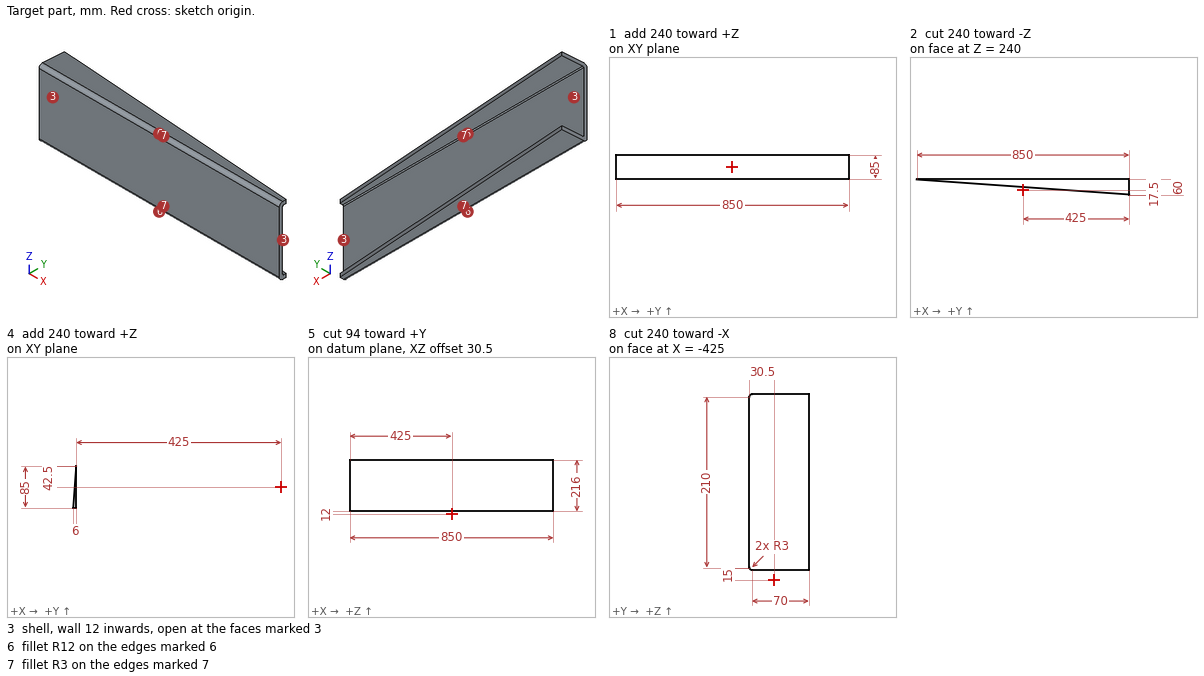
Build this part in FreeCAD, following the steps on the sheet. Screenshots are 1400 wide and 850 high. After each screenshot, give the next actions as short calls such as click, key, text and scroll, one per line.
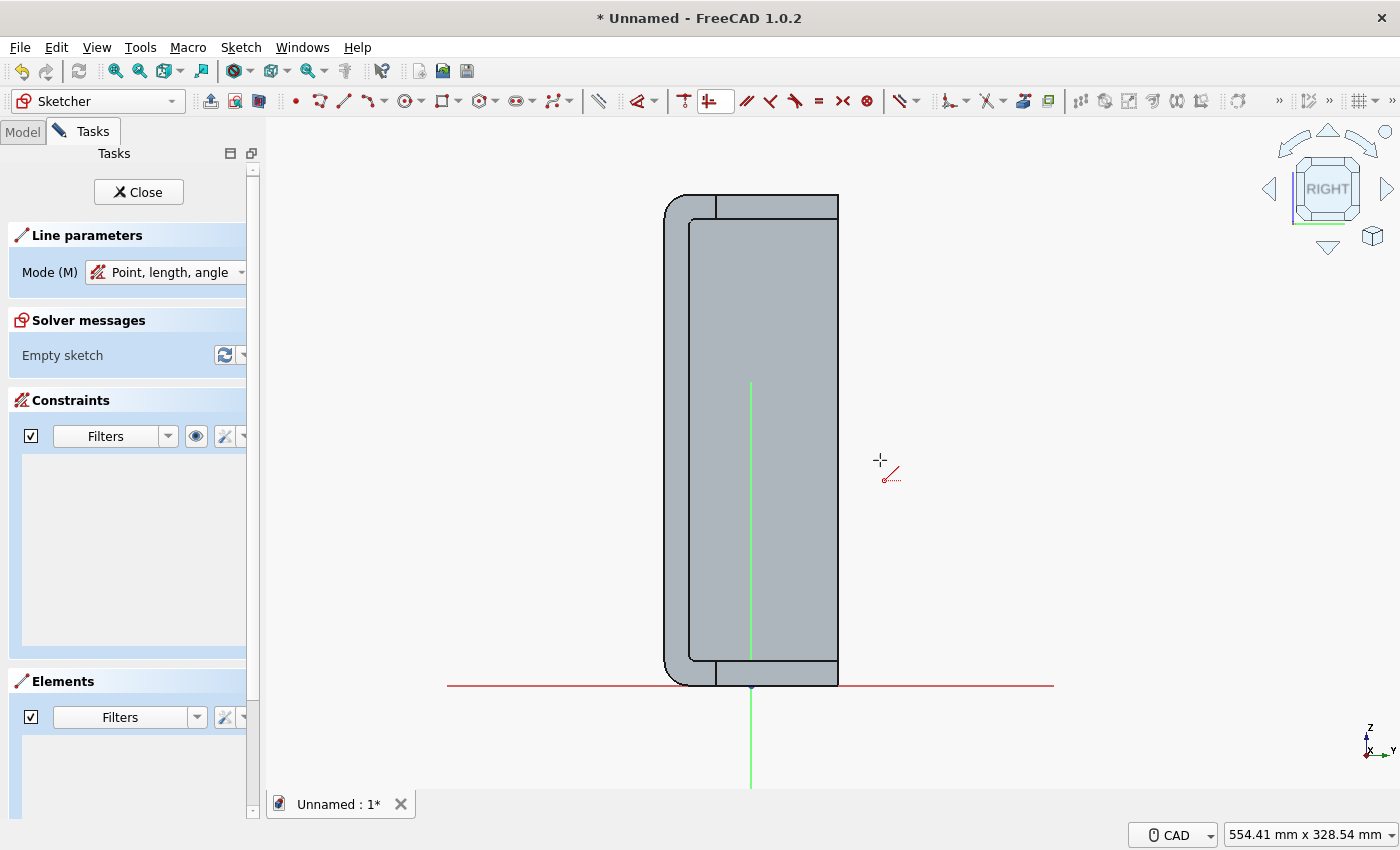
click(689, 225)
click(689, 655)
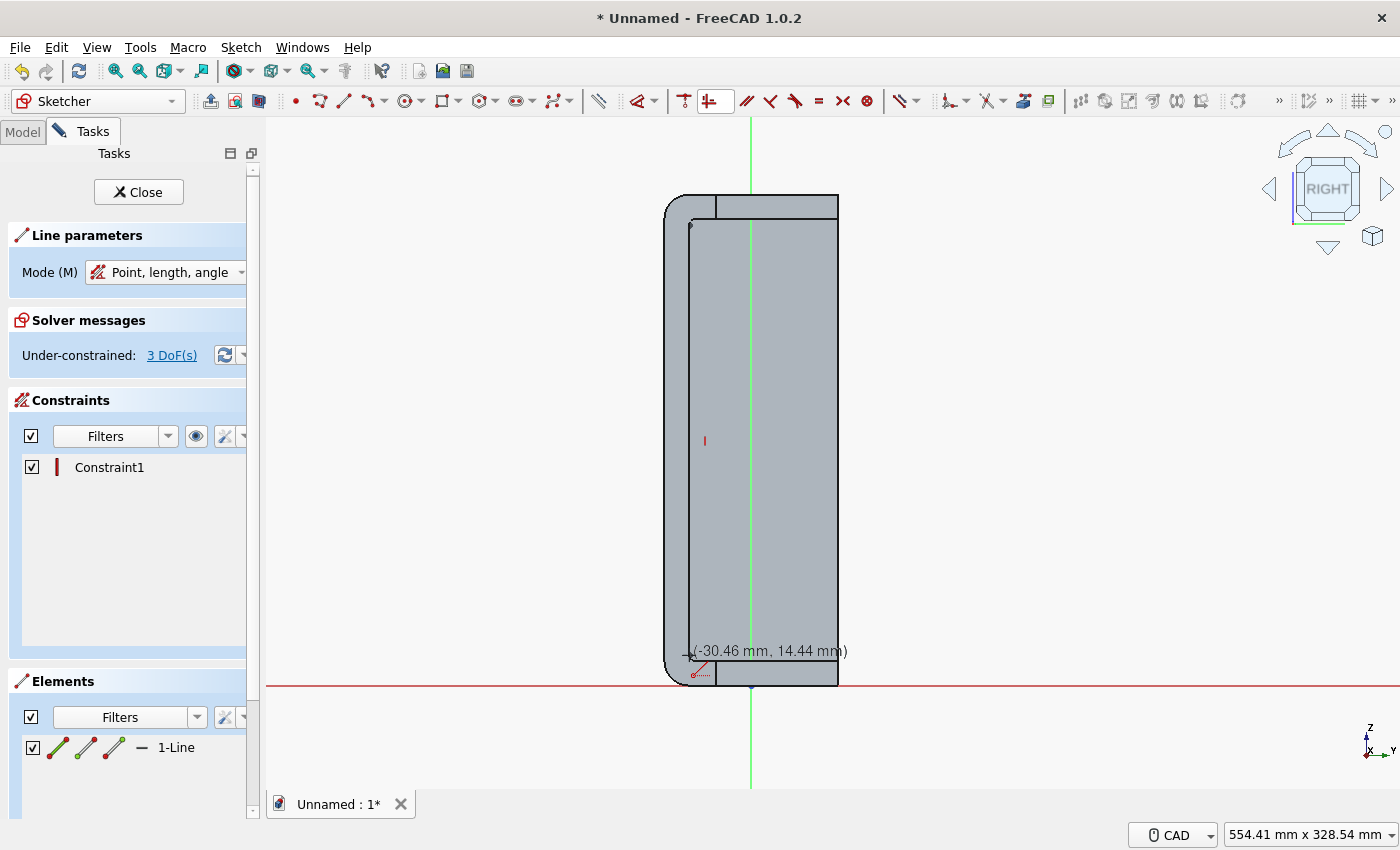
key(g)
key(m)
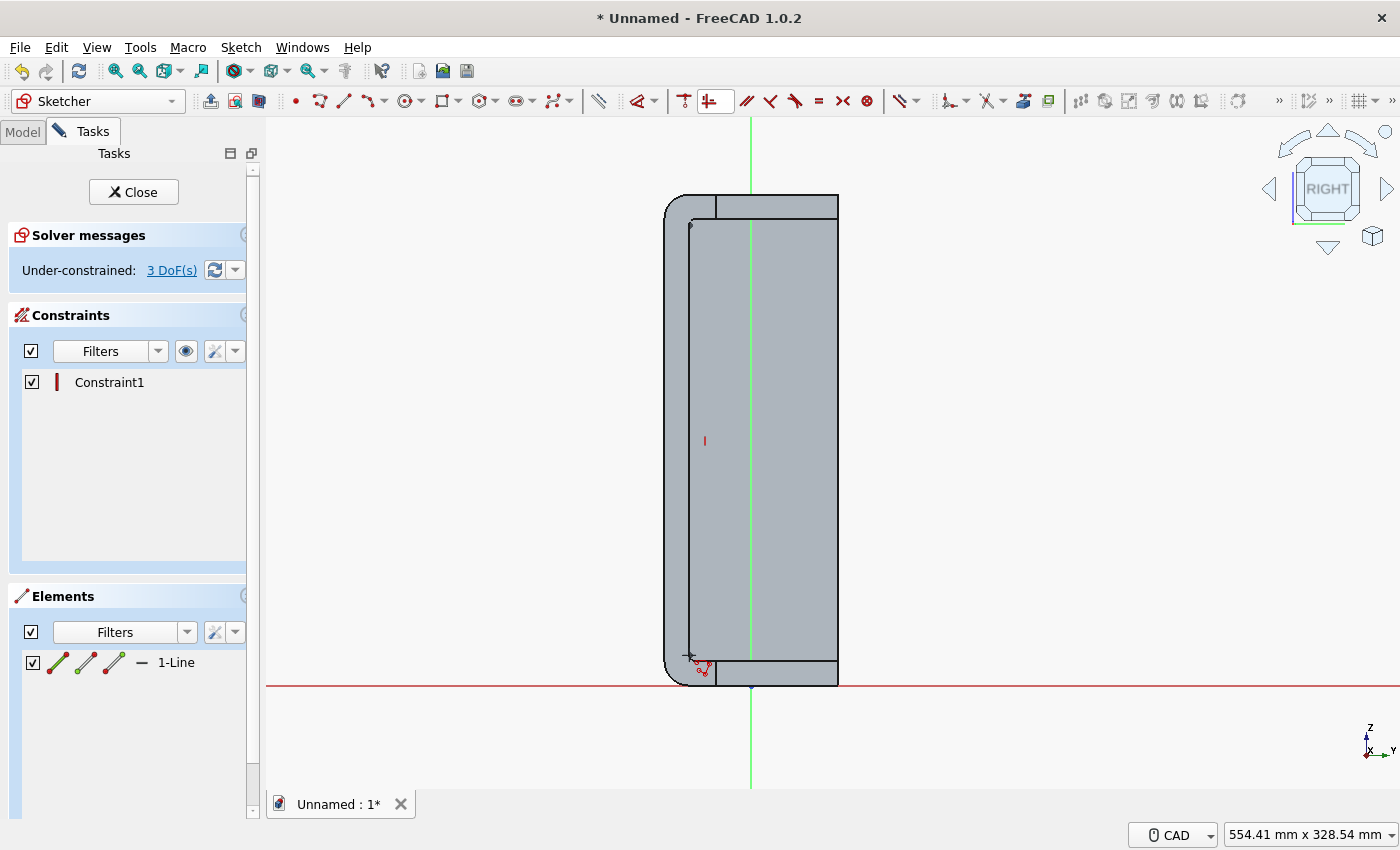
scroll(695, 661, up, 4)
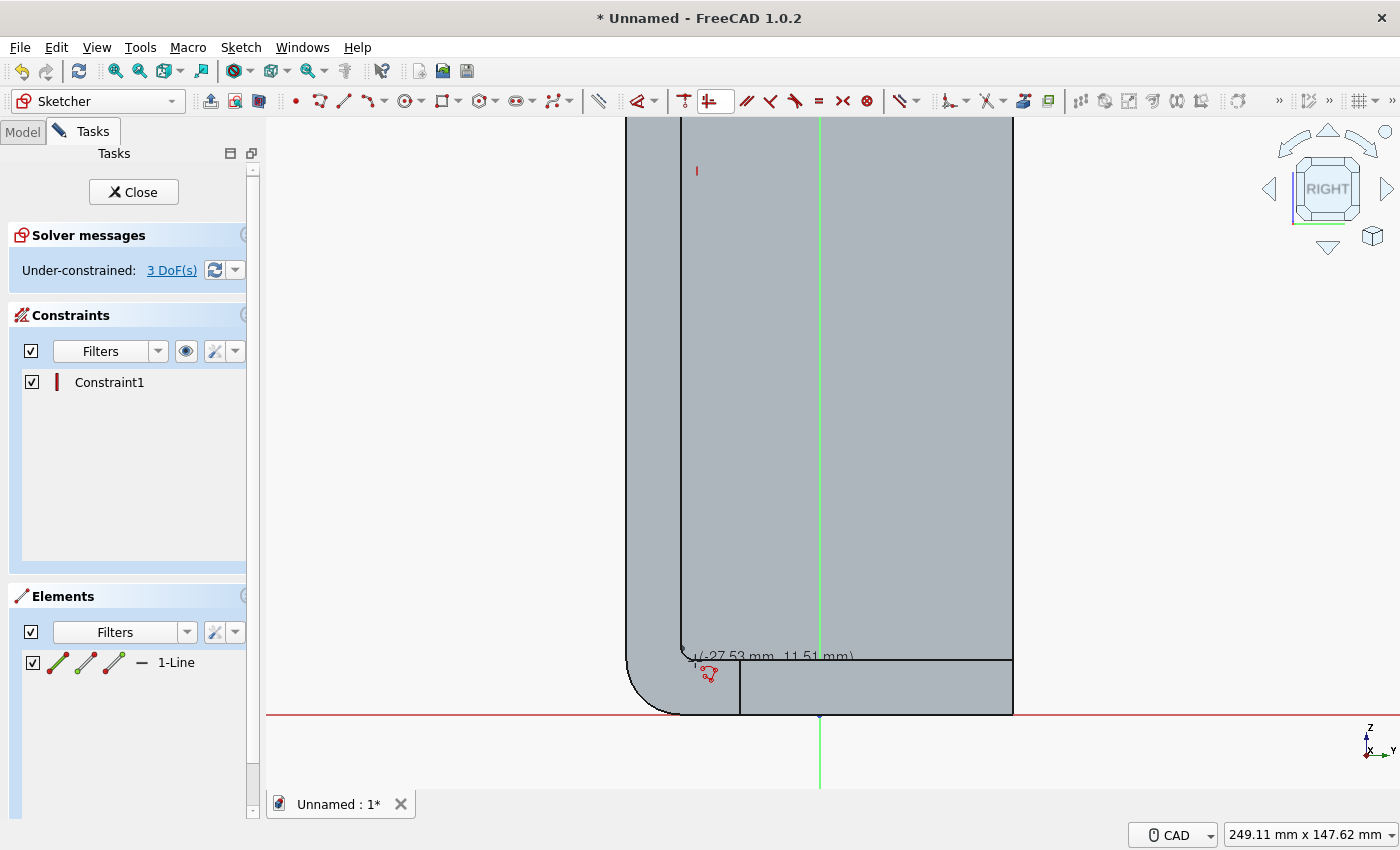
click(695, 660)
click(1013, 660)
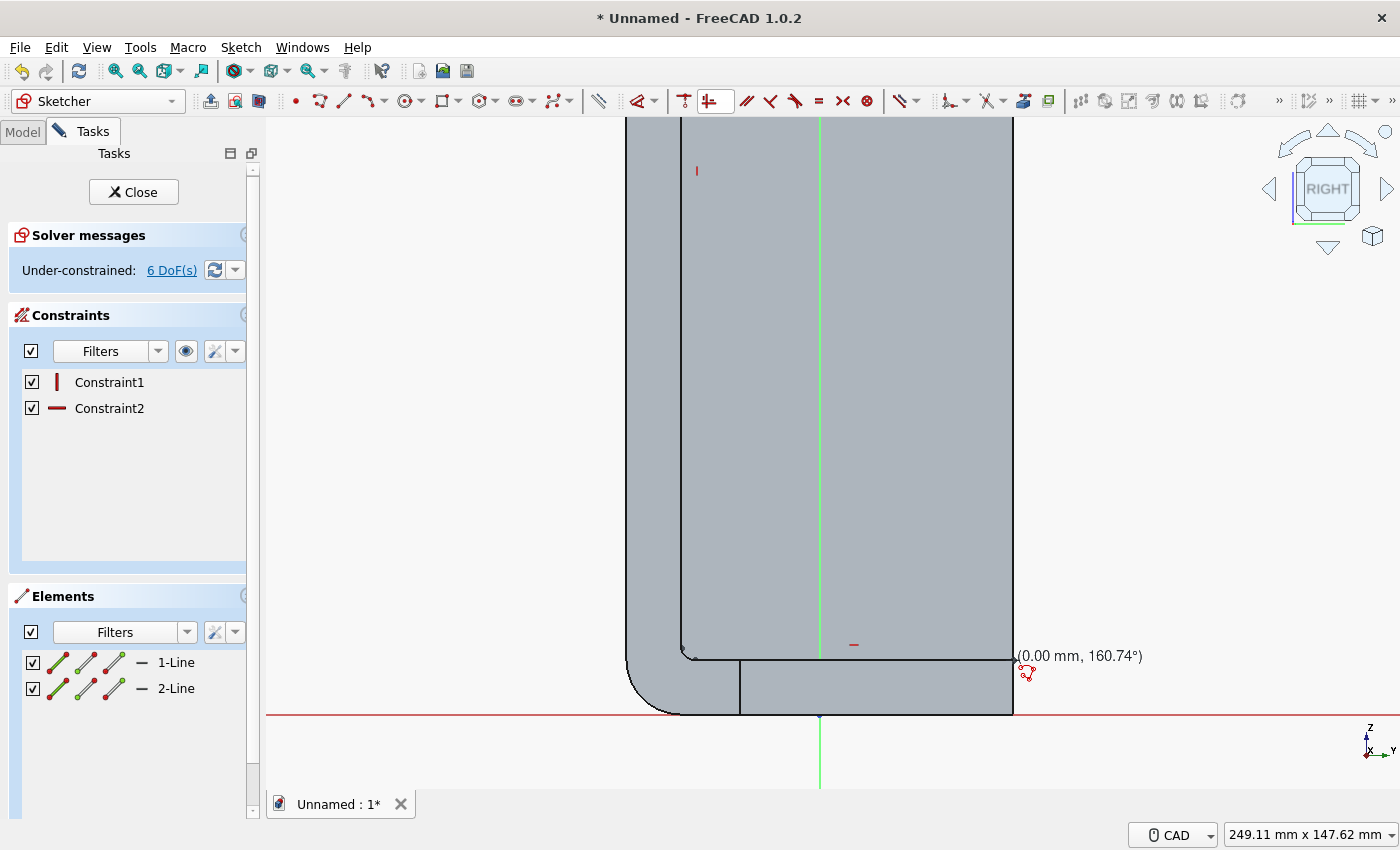
scroll(697, 663, down, 4)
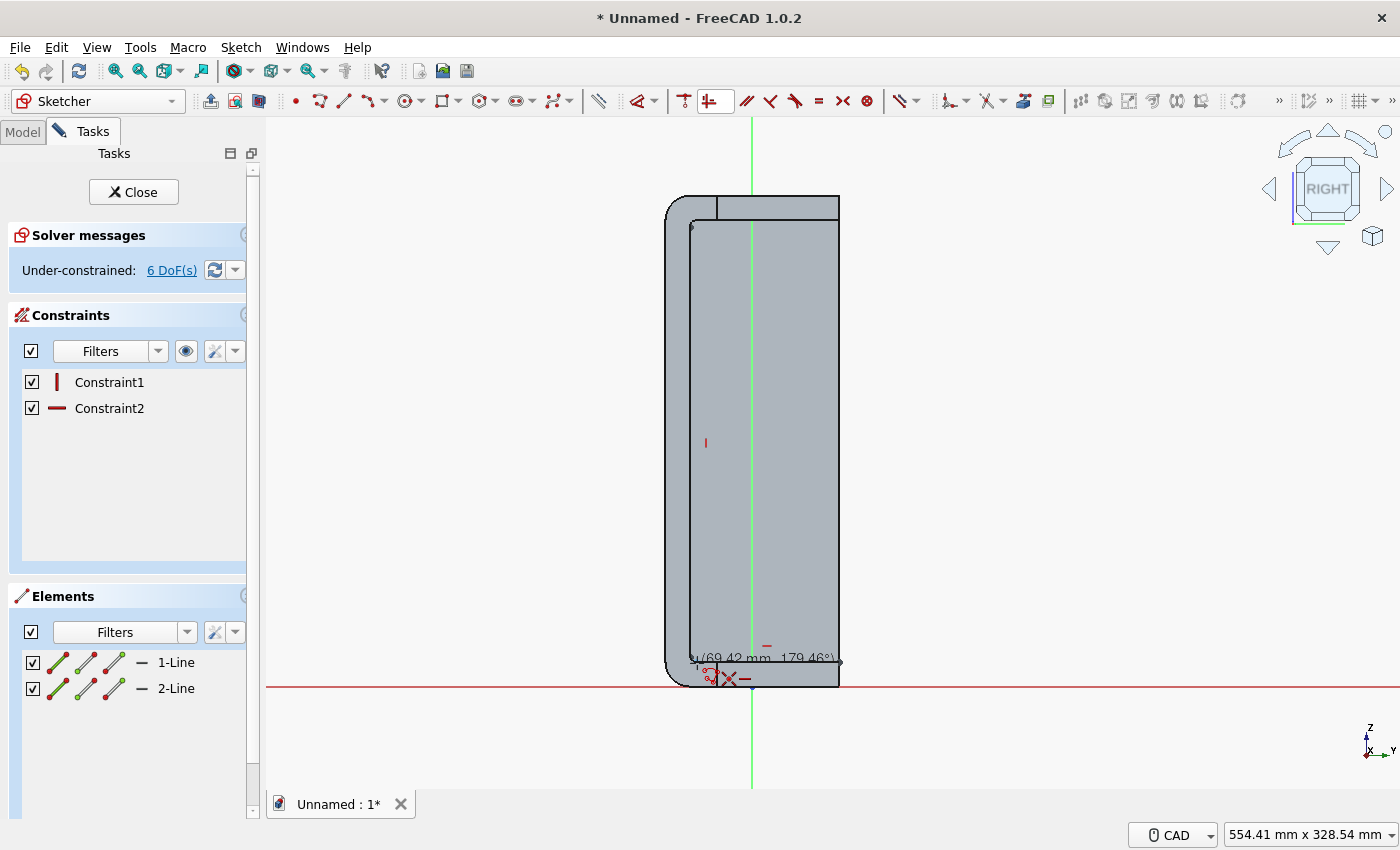
click(839, 220)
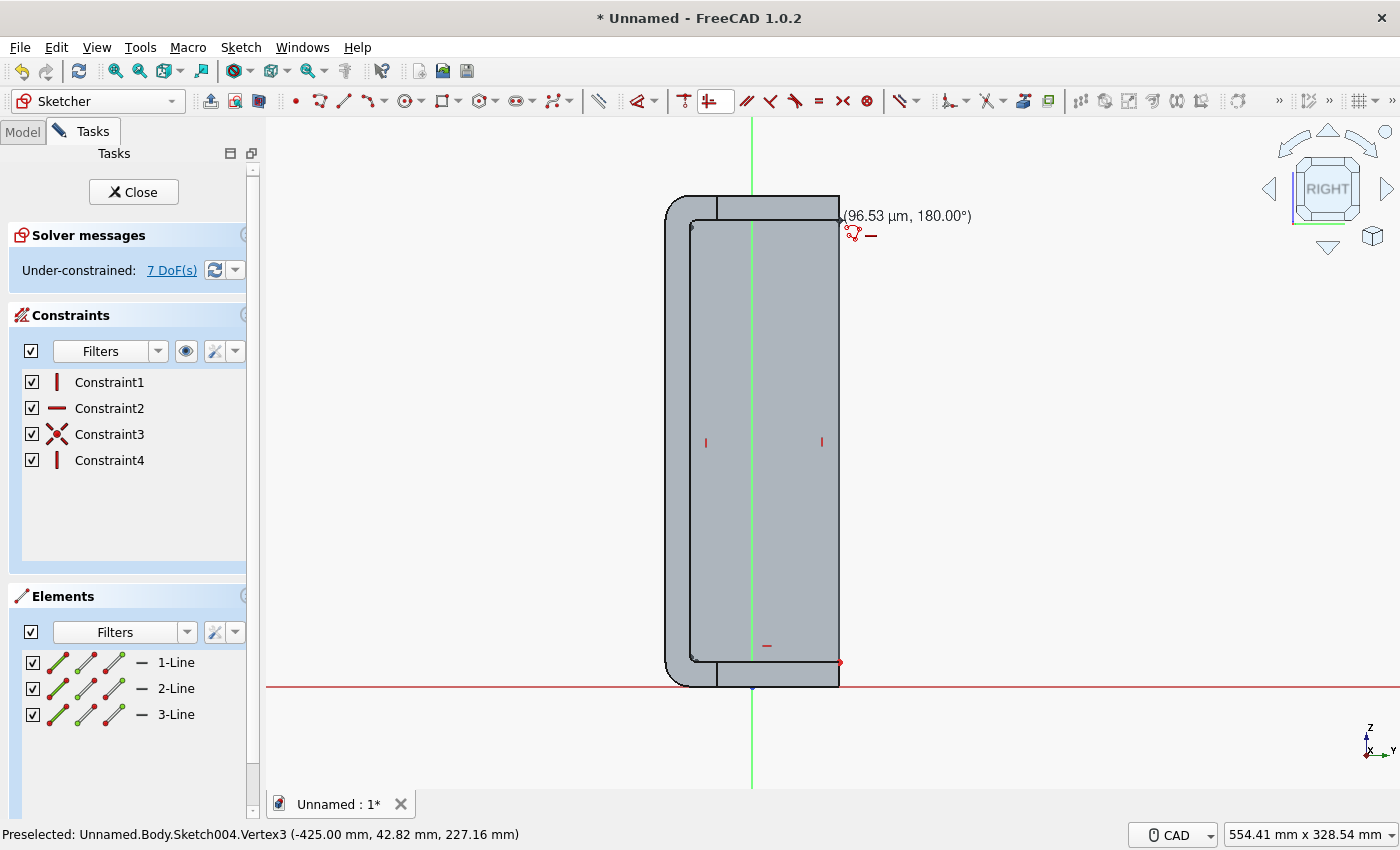
scroll(696, 220, up, 4)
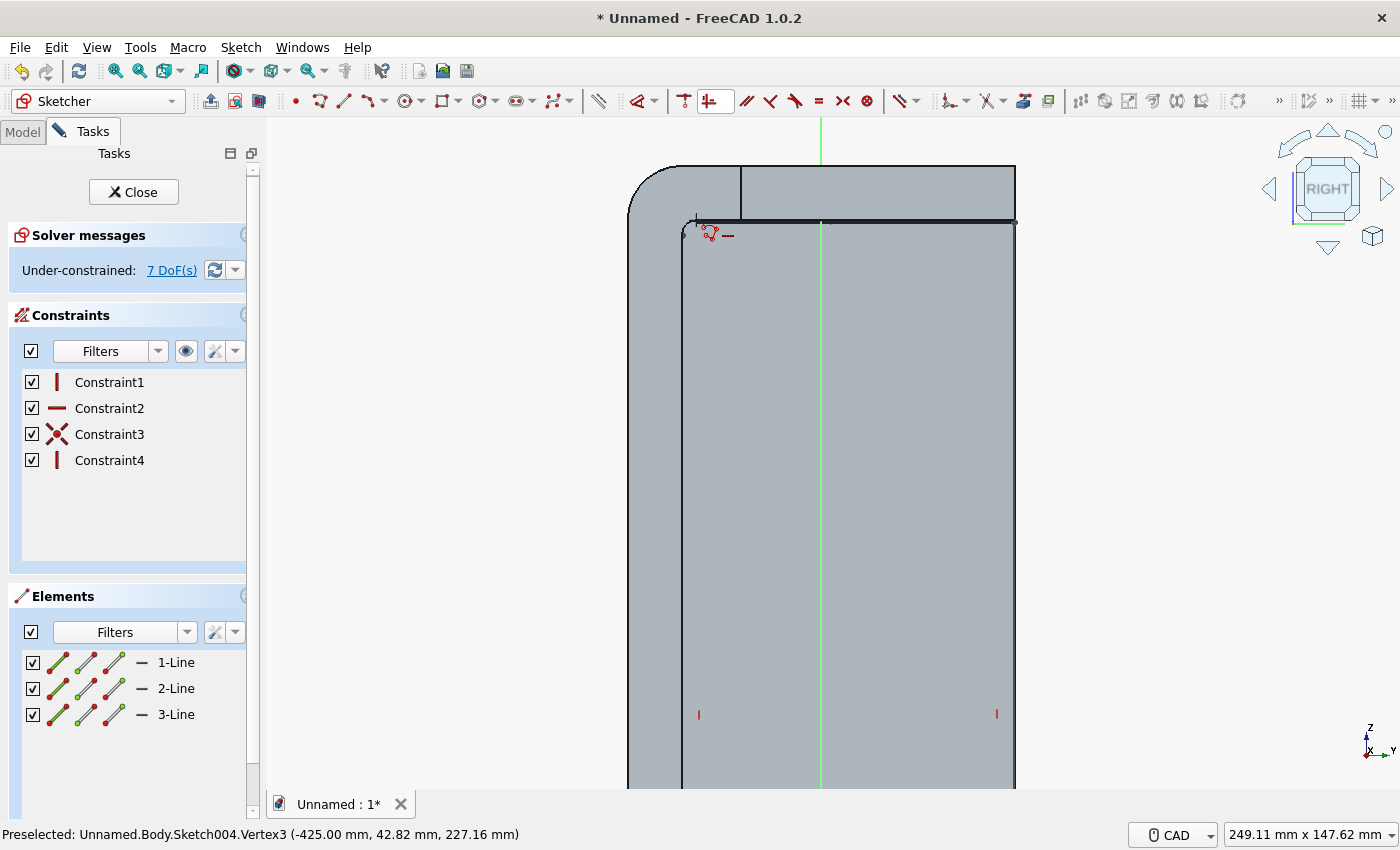
click(696, 220)
right_click(696, 220)